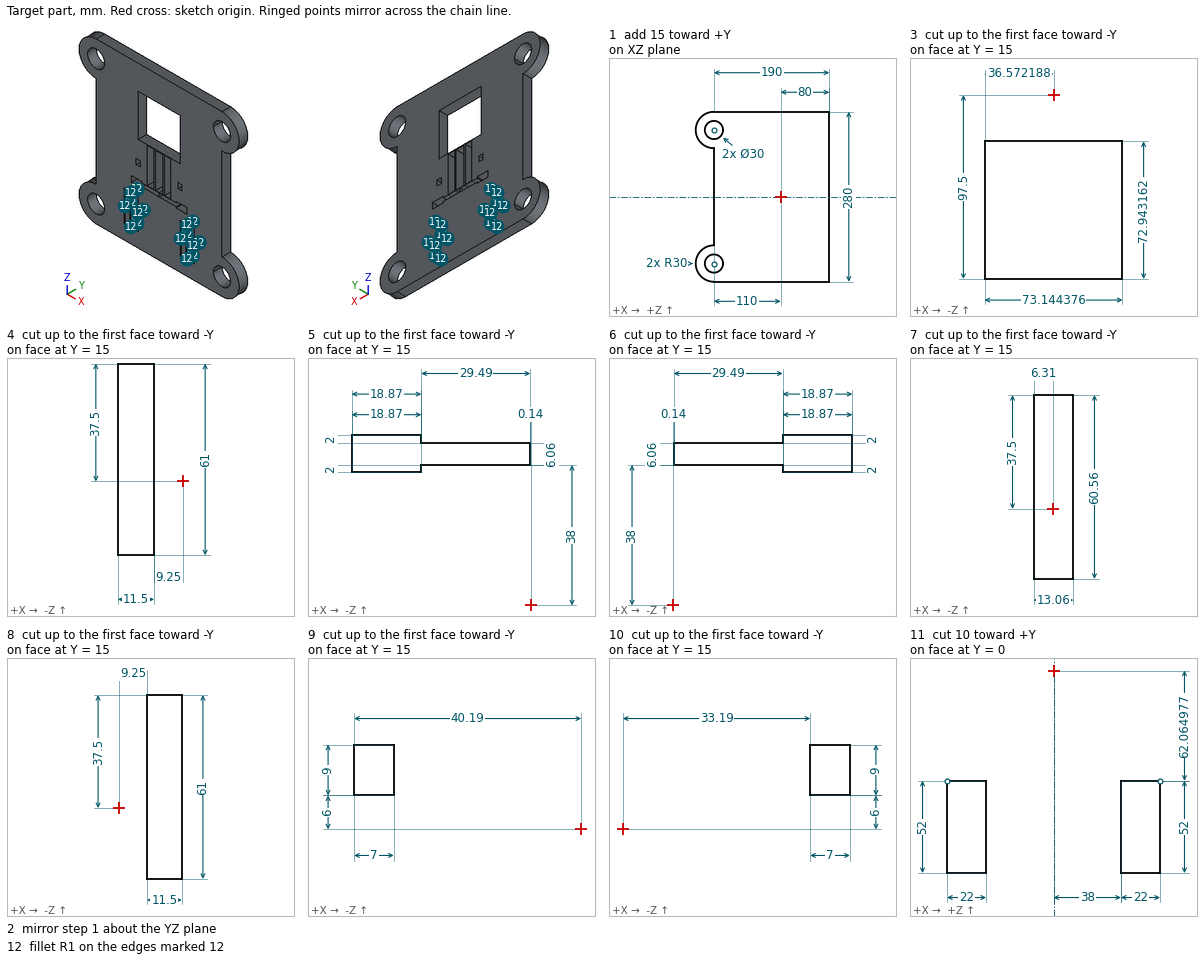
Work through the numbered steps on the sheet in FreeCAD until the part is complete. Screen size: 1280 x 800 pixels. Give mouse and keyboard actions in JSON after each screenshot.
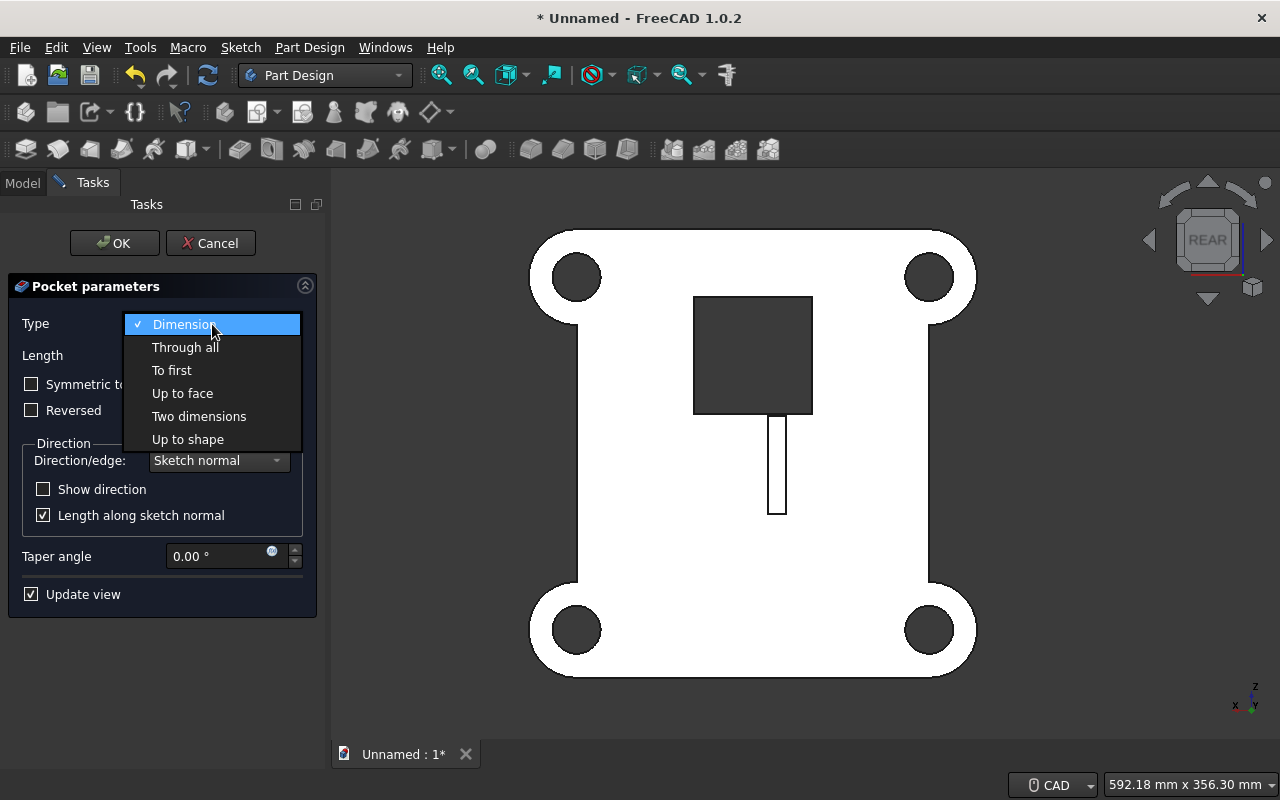
{"action": "left_click", "coordinate": [212, 370]}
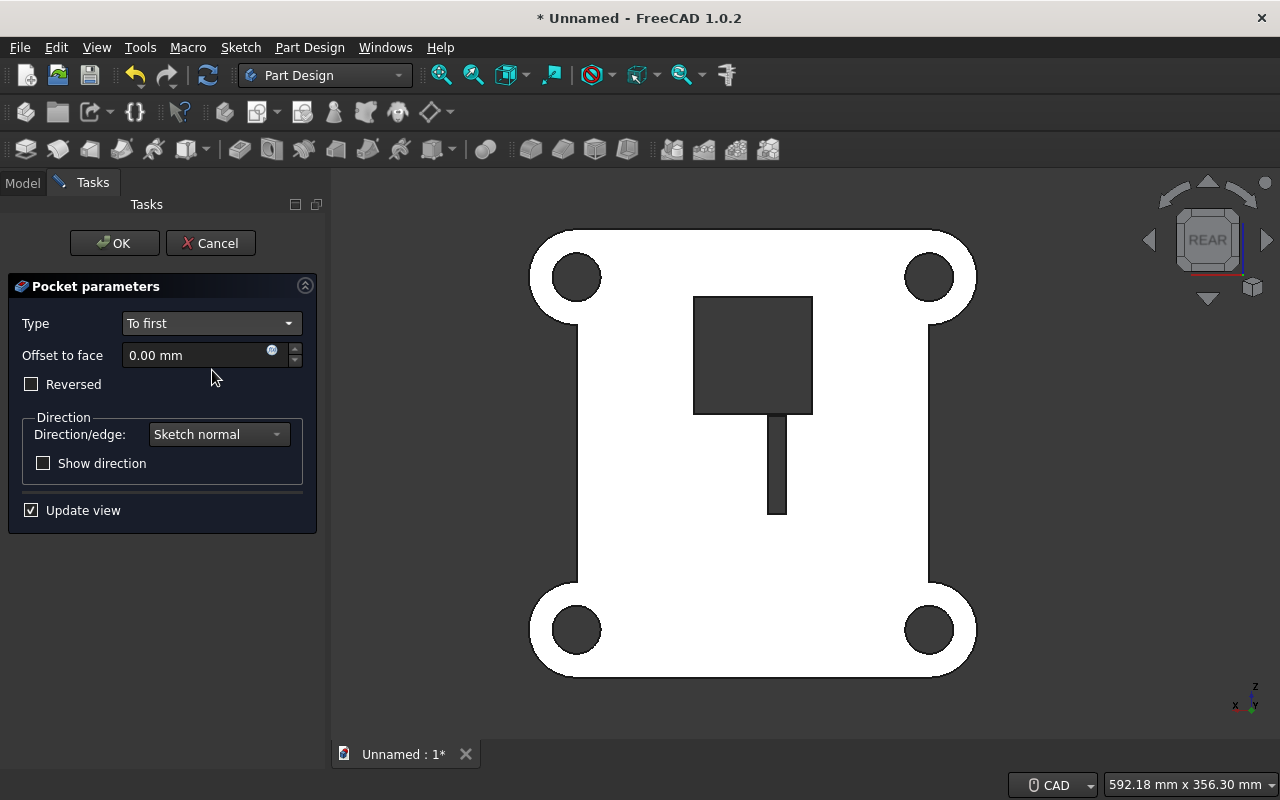
{"action": "left_click", "coordinate": [115, 243]}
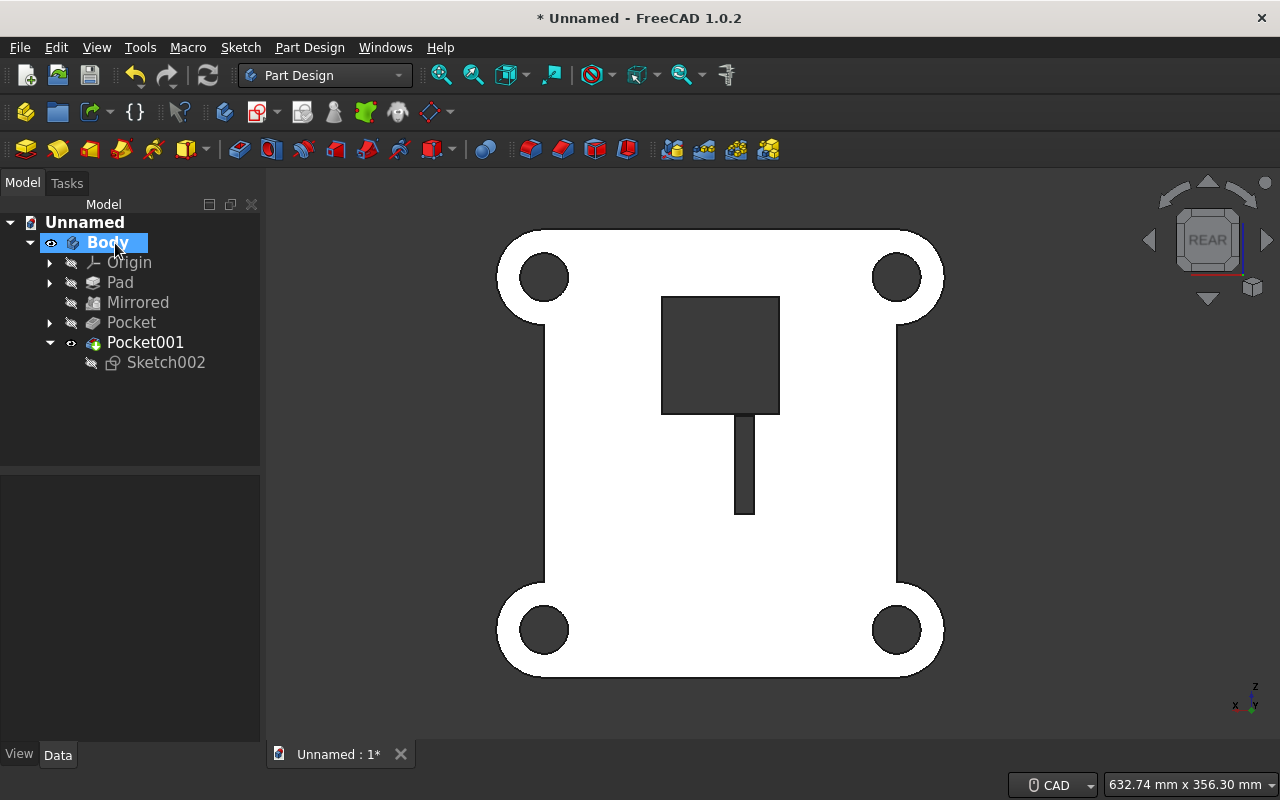
{"action": "left_click", "coordinate": [656, 581]}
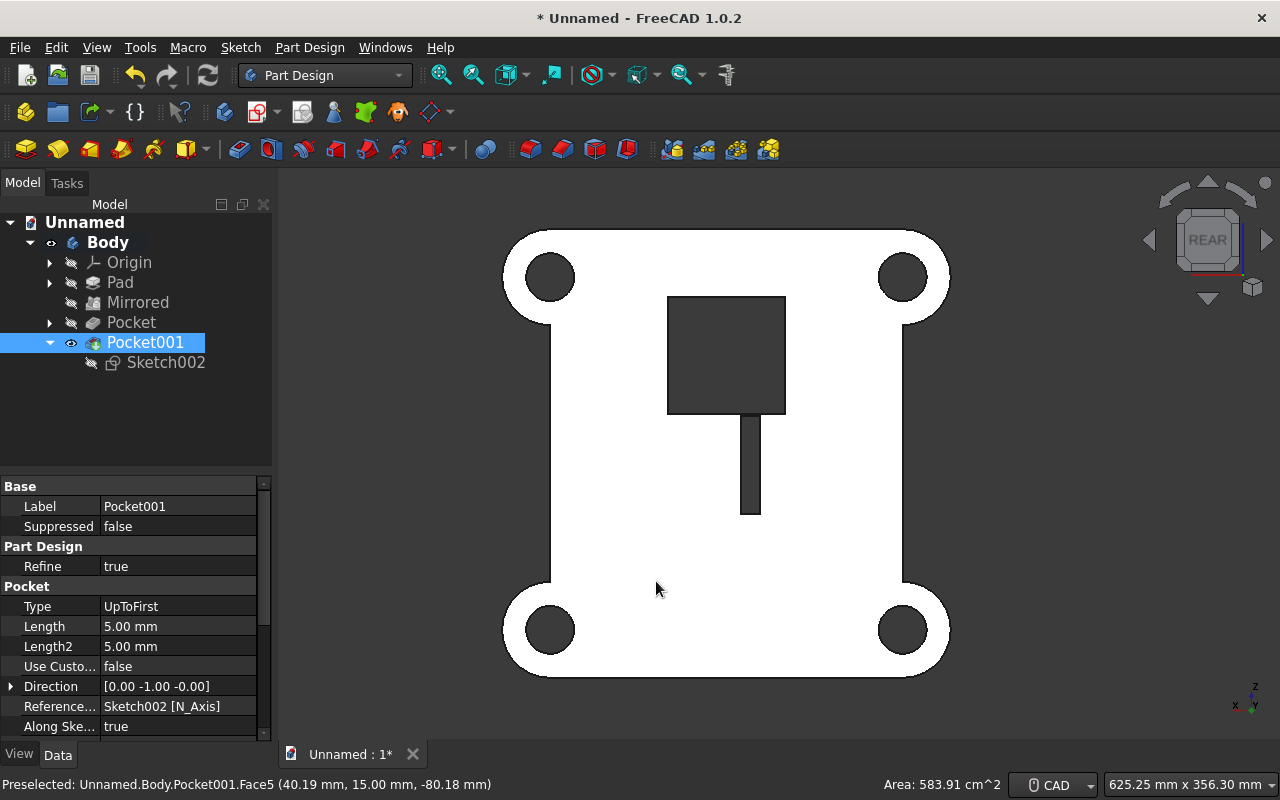
{"action": "left_click", "coordinate": [258, 112]}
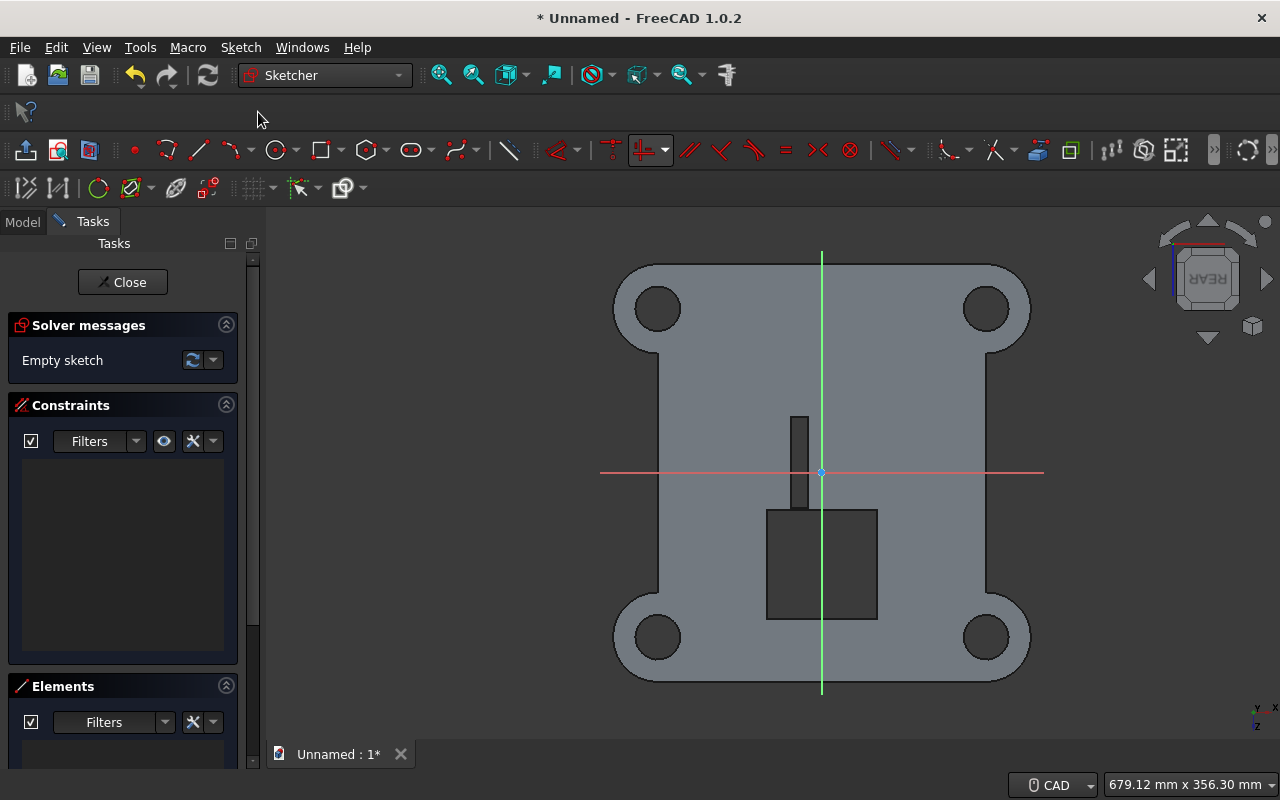
{"action": "scroll", "coordinate": [806, 430], "scroll_direction": "up", "scroll_amount": 8}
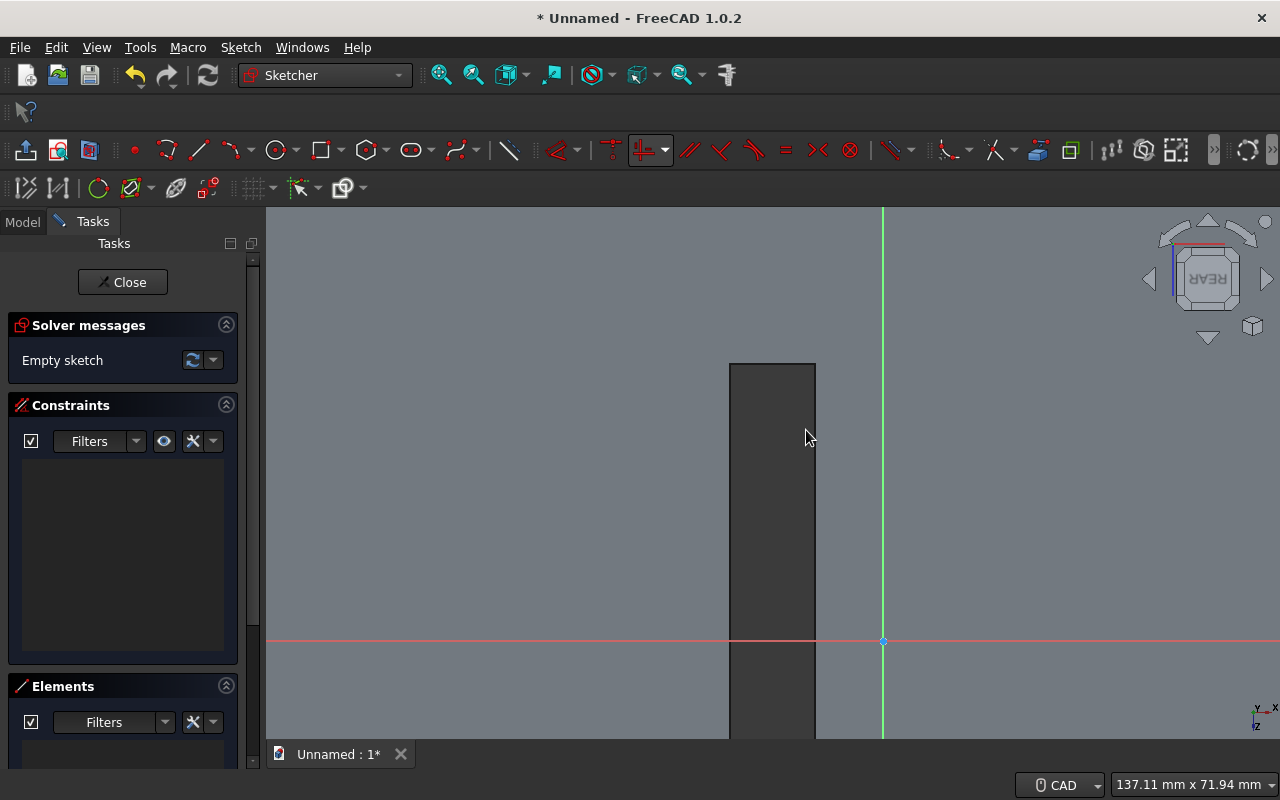
{"action": "key", "text": "g m"}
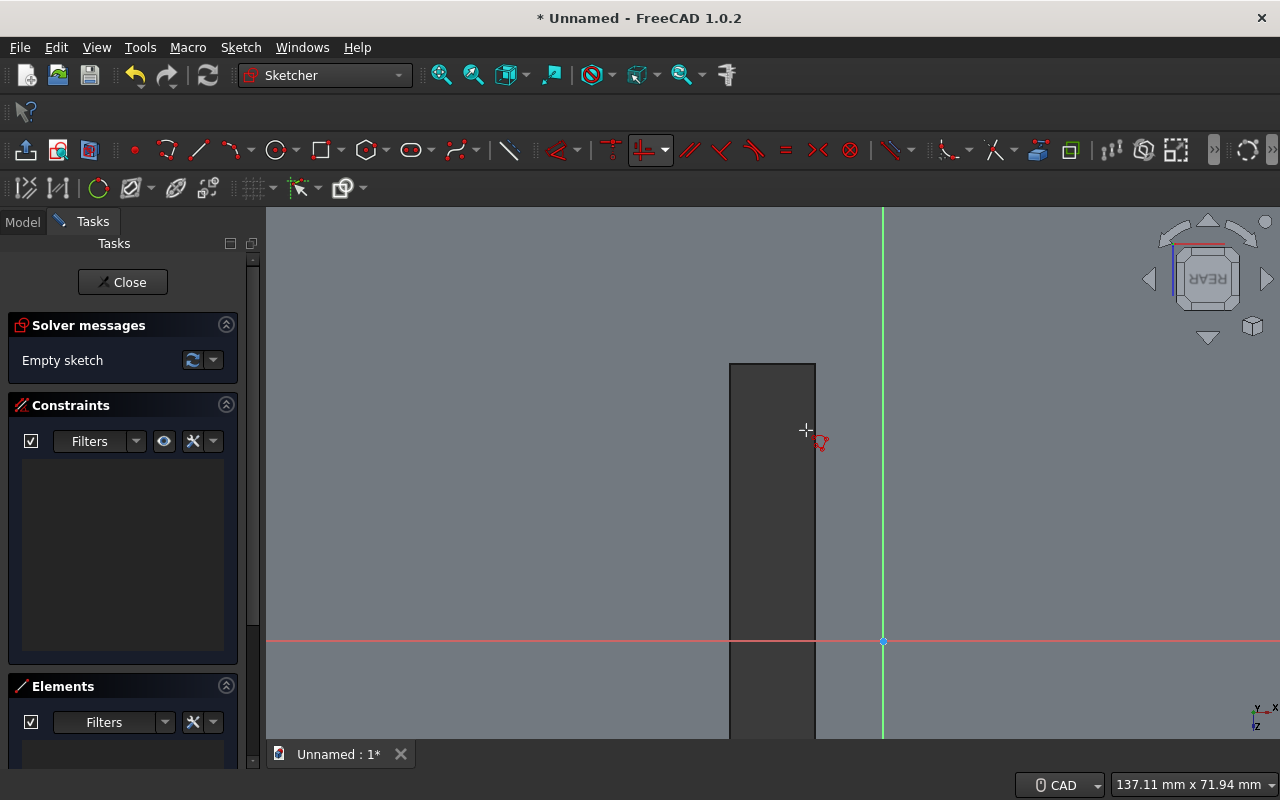
{"action": "scroll", "coordinate": [882, 360], "scroll_direction": "up", "scroll_amount": 14}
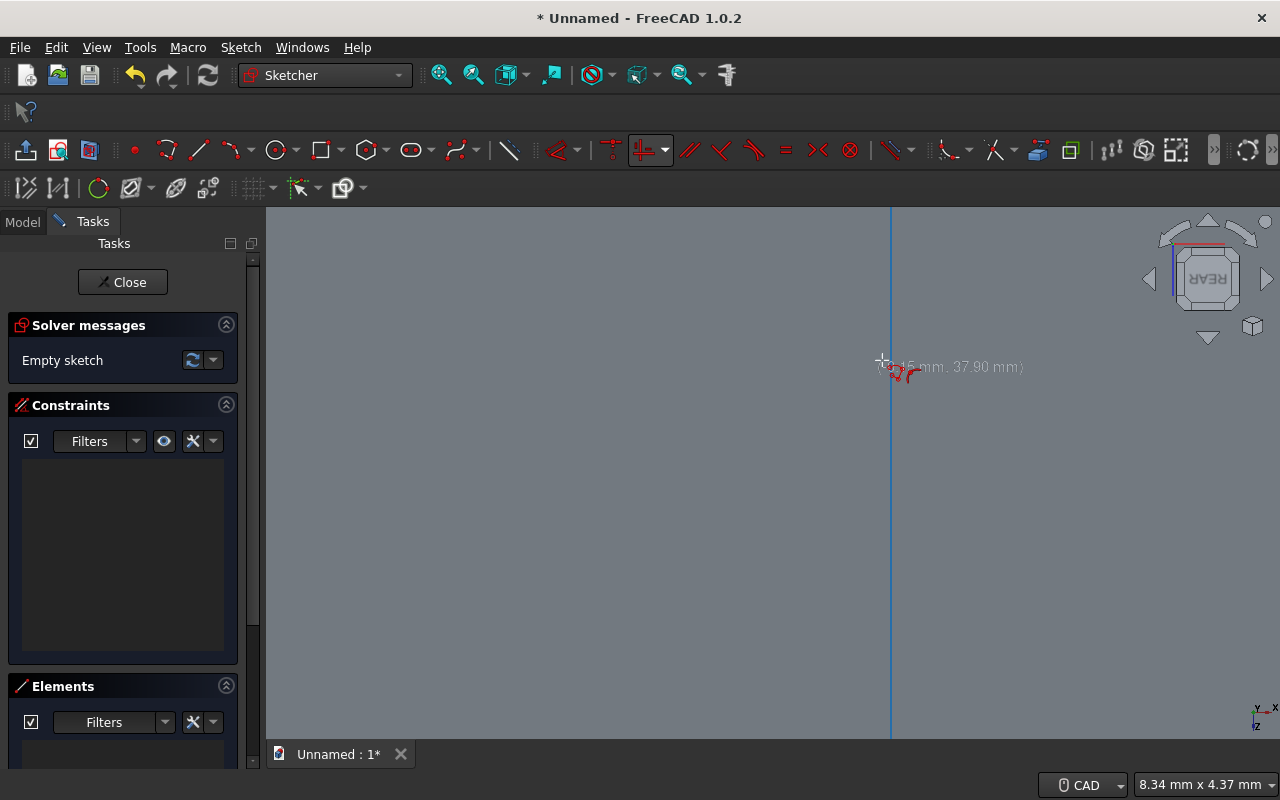
{"action": "left_click", "coordinate": [874, 360]}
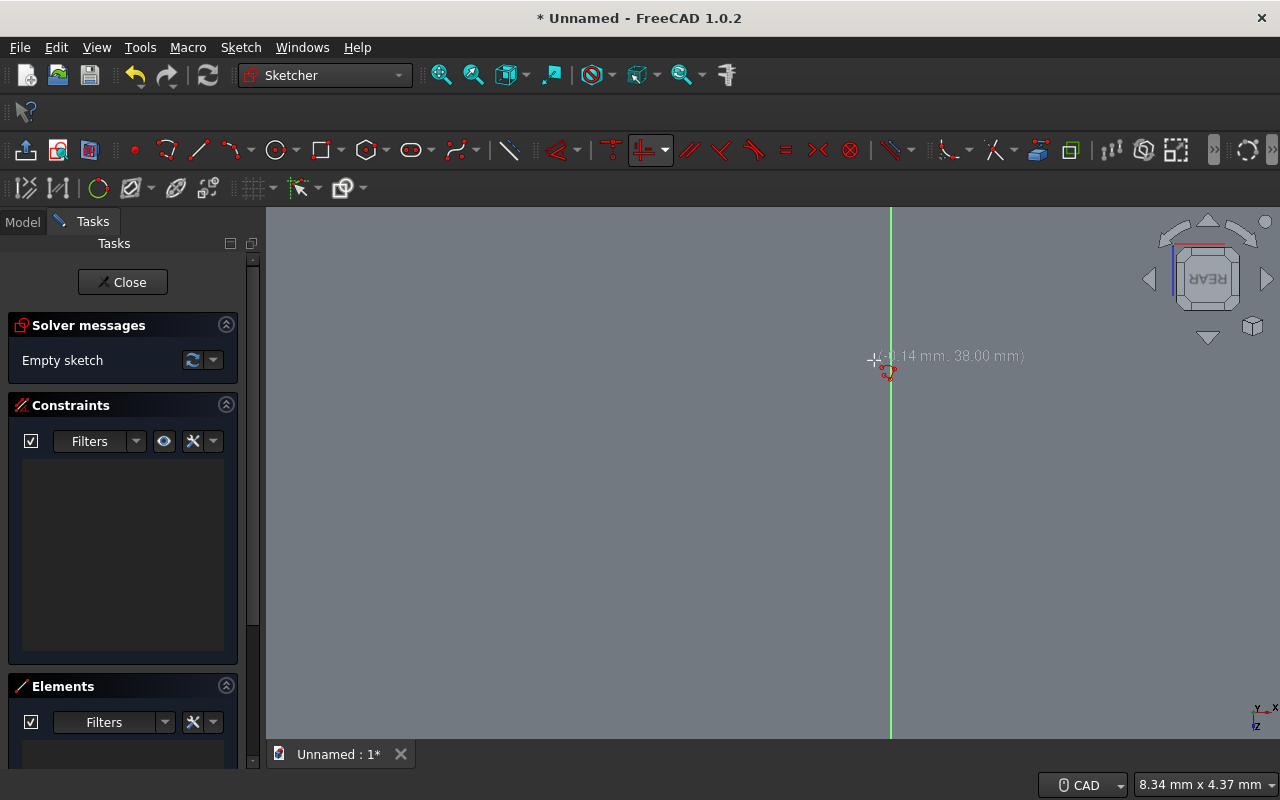
{"action": "scroll", "coordinate": [883, 362], "scroll_direction": "down", "scroll_amount": 14}